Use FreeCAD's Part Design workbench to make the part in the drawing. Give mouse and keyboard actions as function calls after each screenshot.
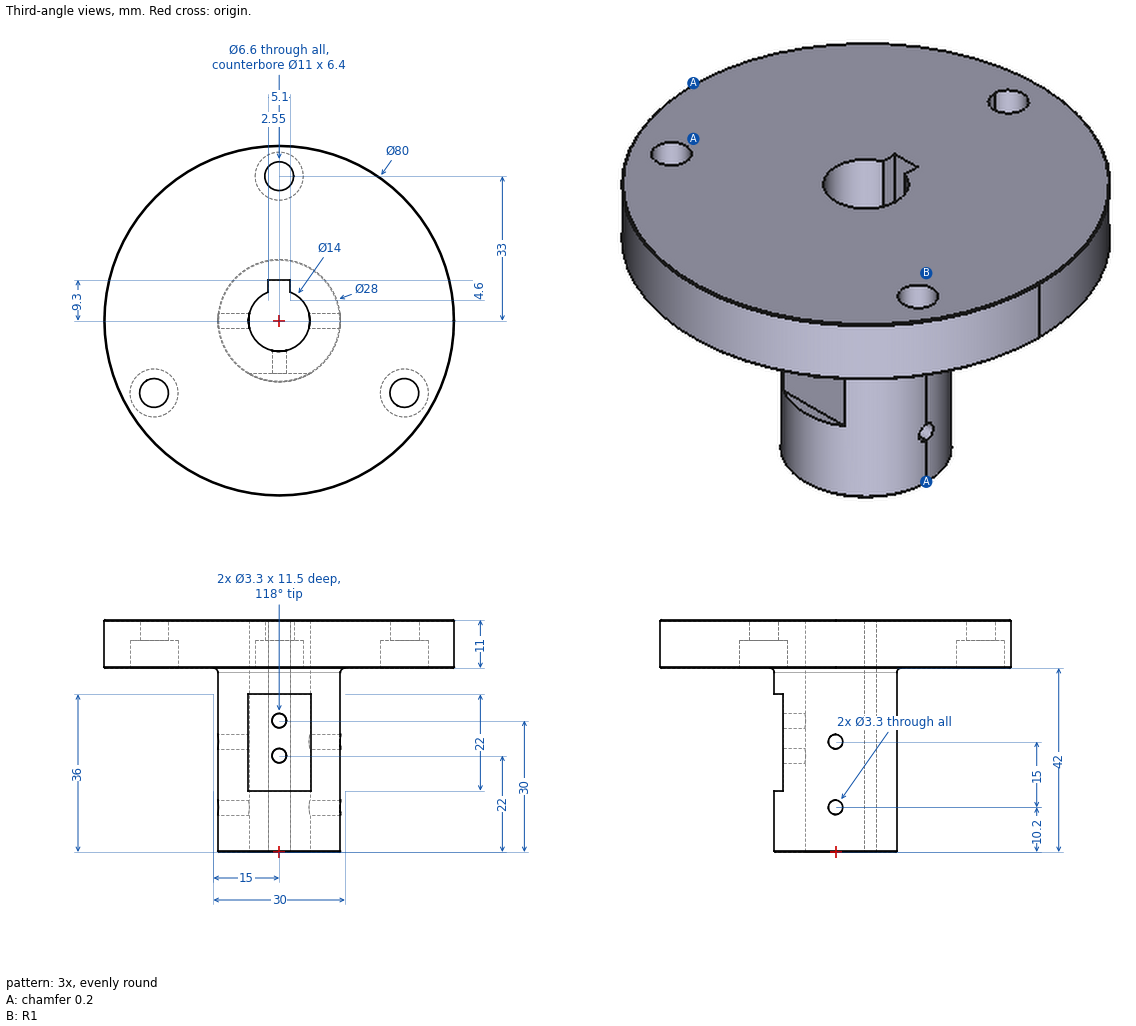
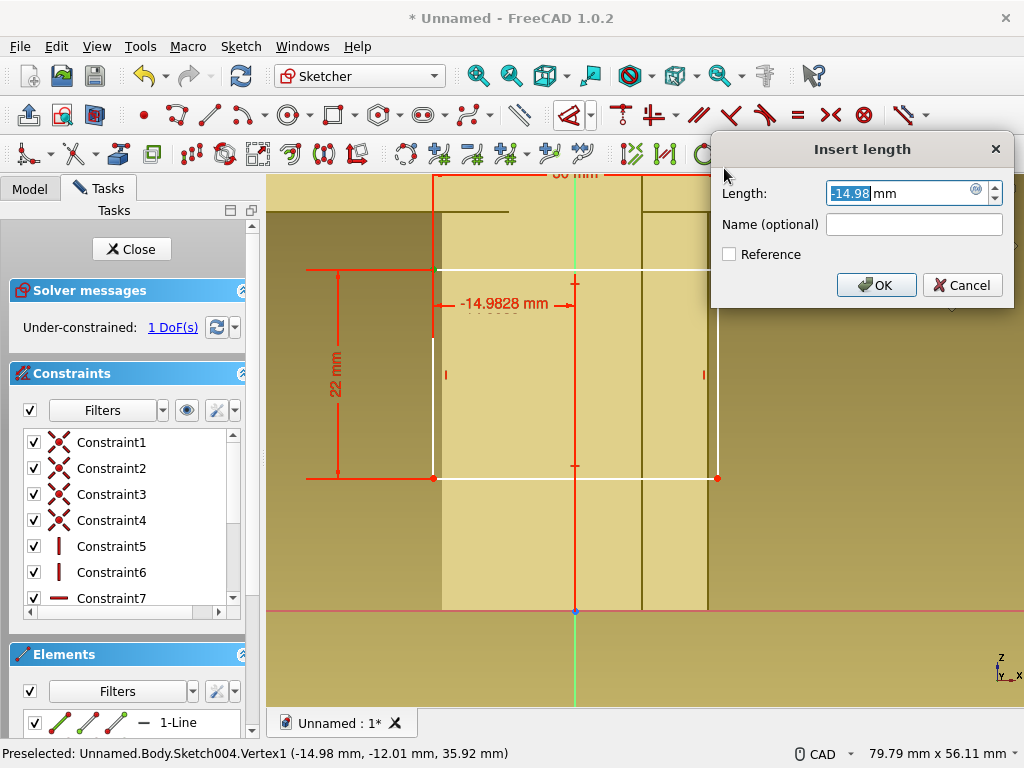
text(-15)
key(Return)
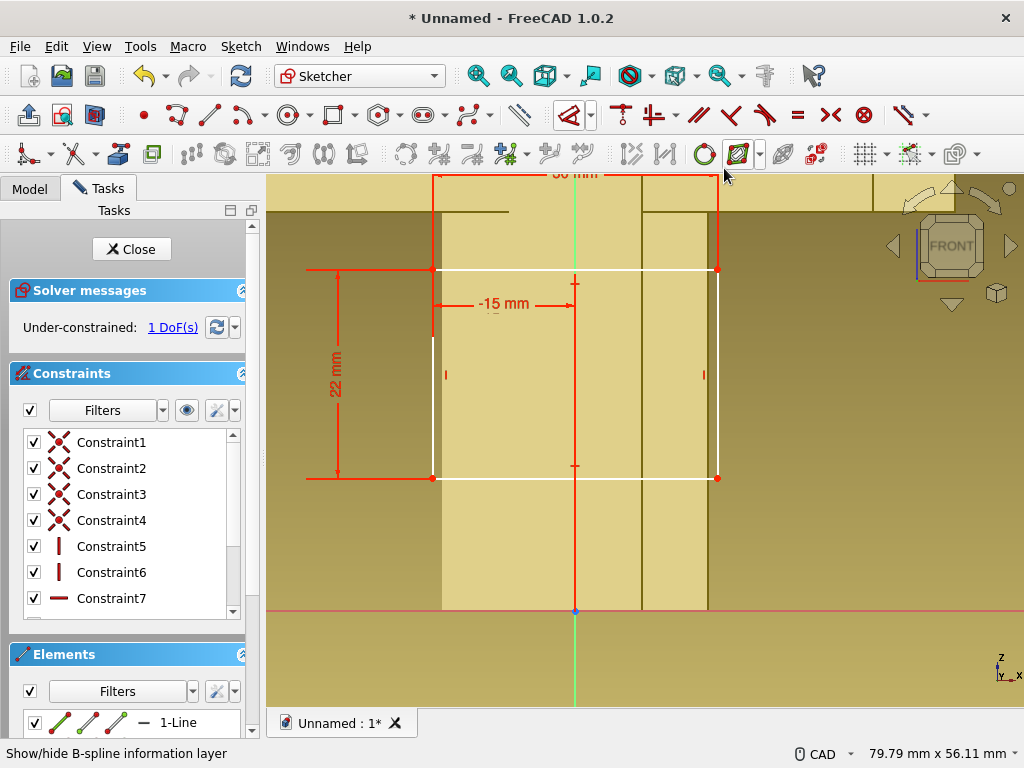
click(433, 270)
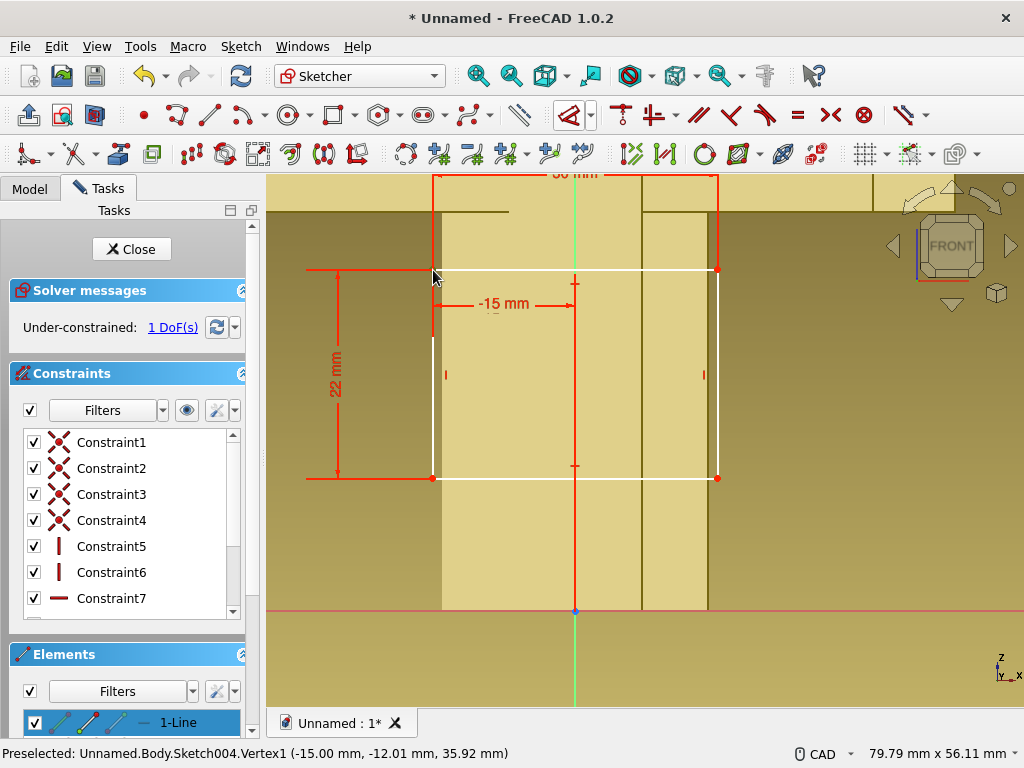
key(i)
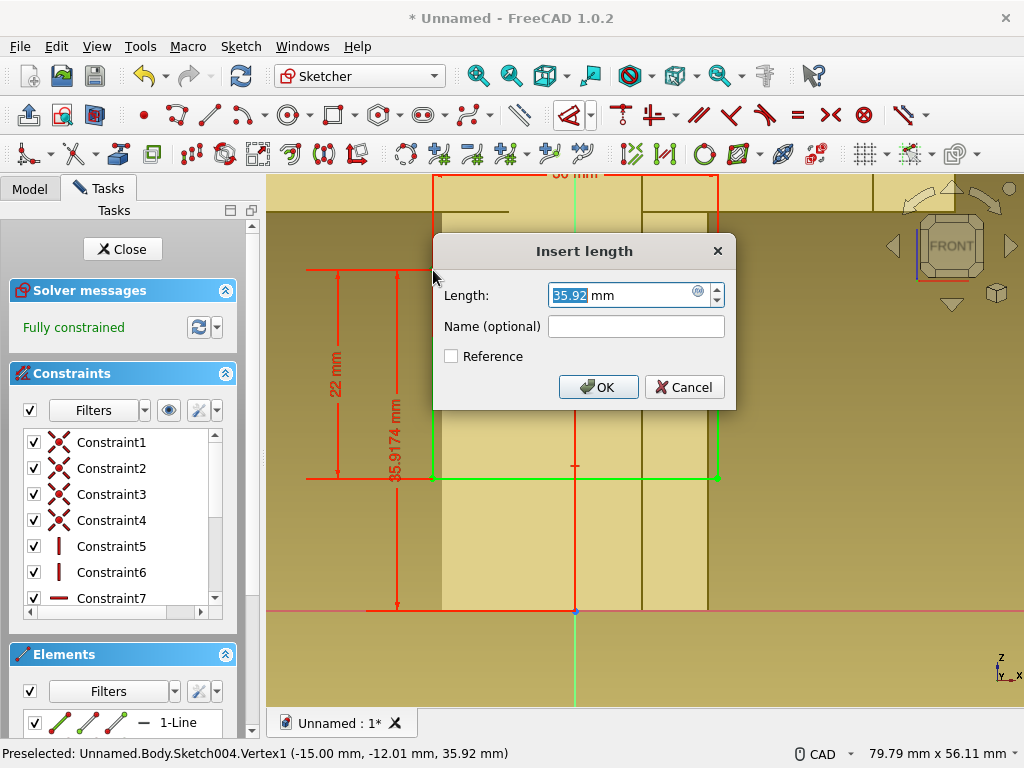
text(36)
key(Return)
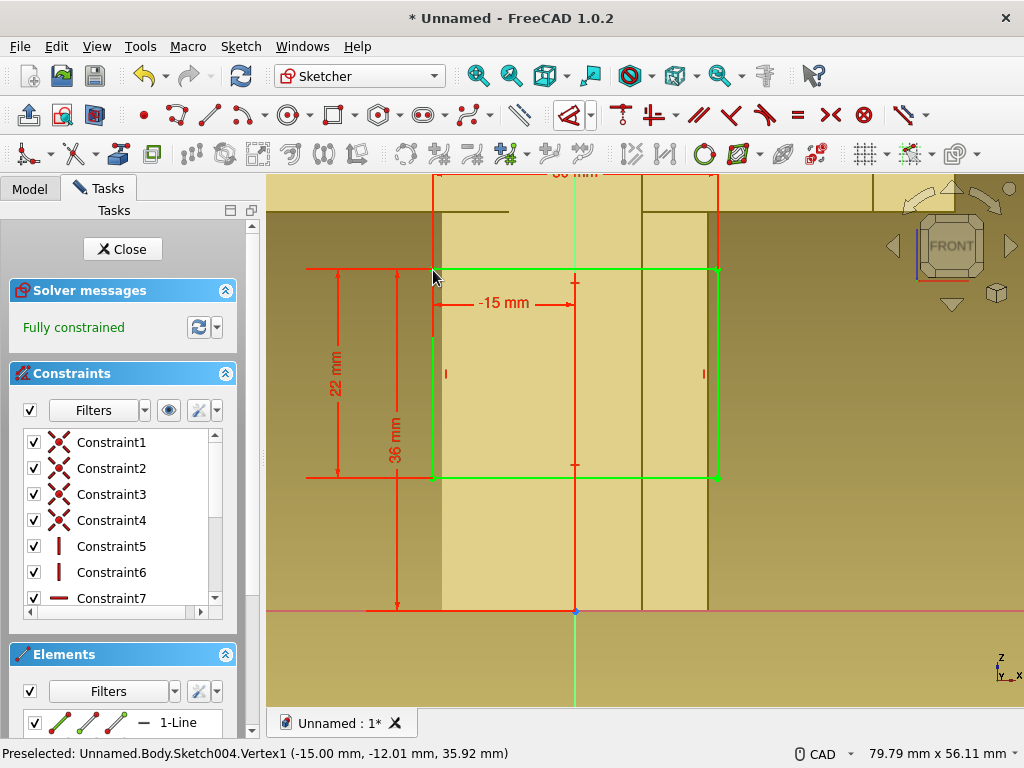
click(123, 249)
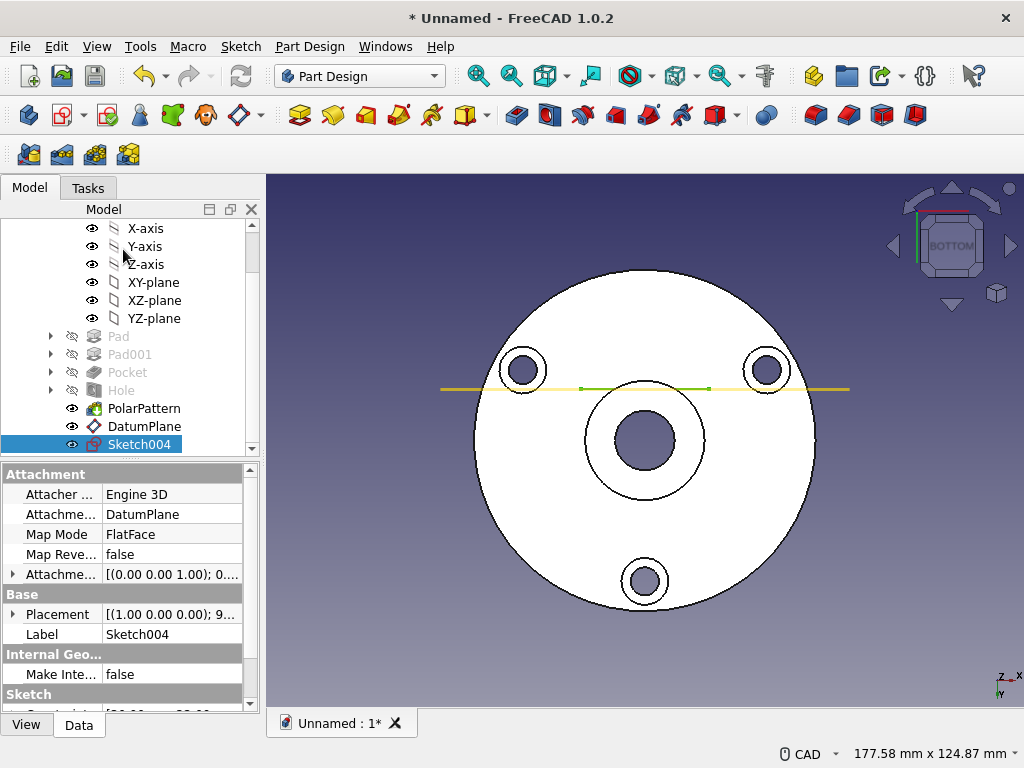
click(517, 116)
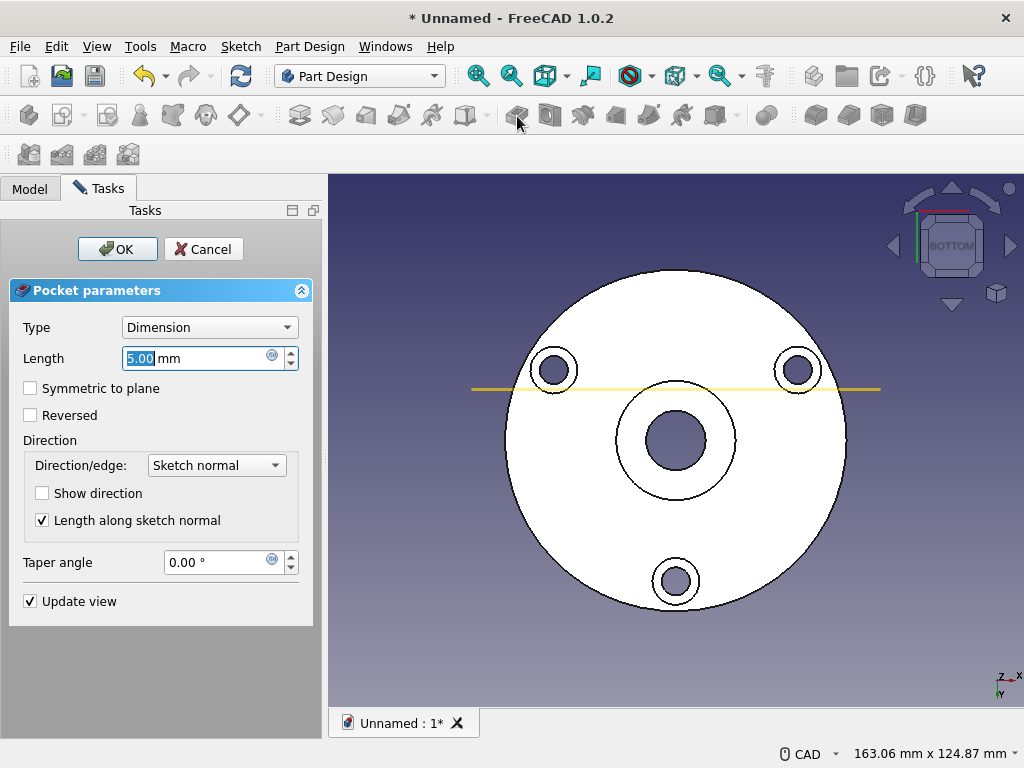
click(210, 328)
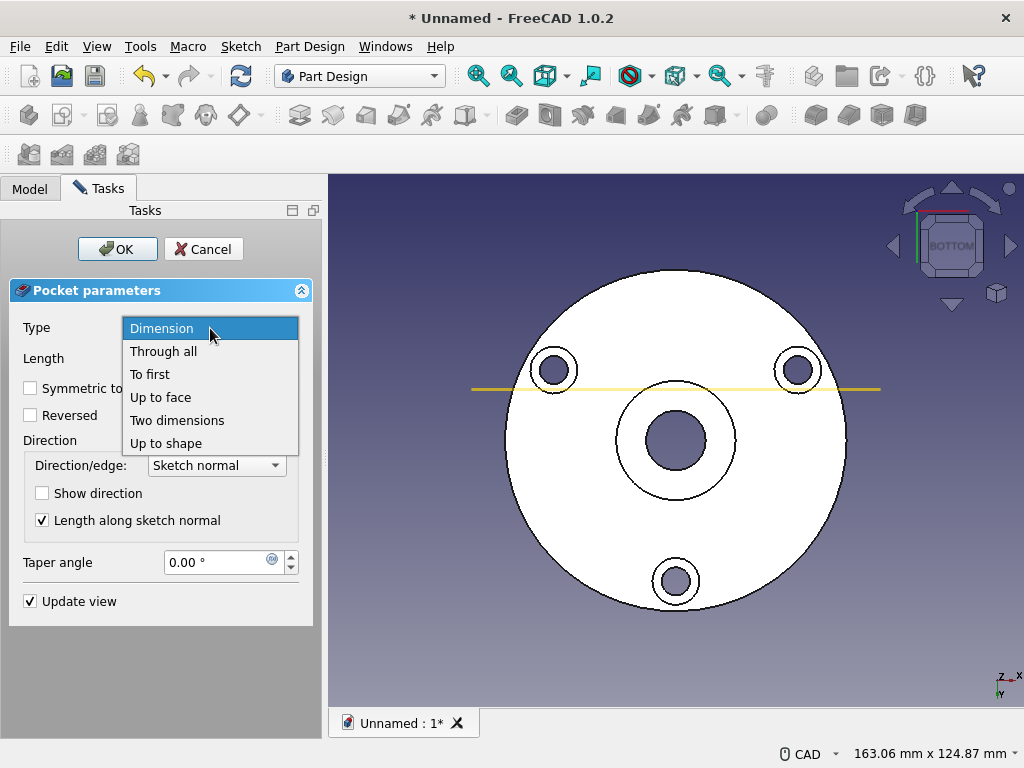
click(208, 352)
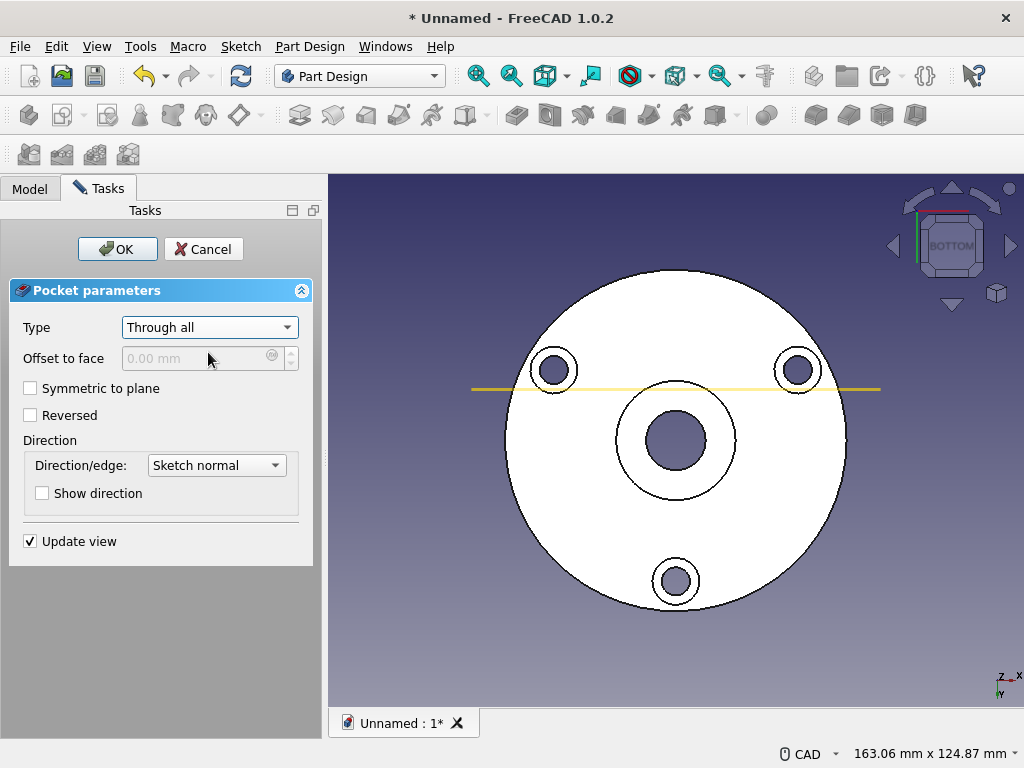
click(31, 415)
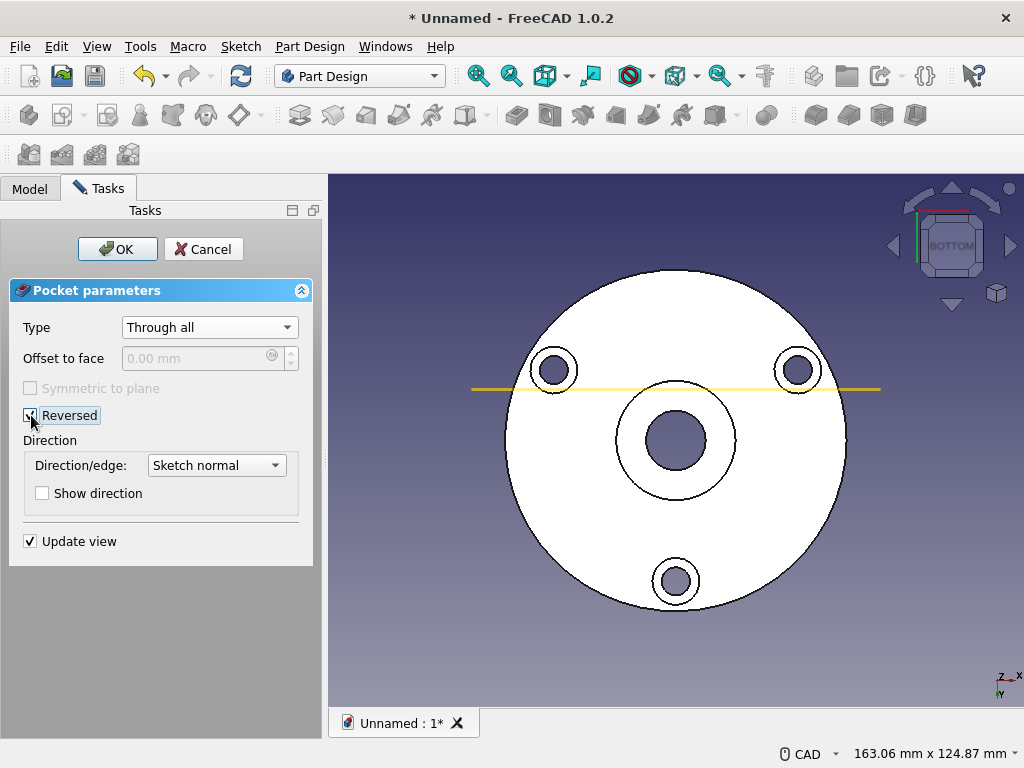
click(118, 249)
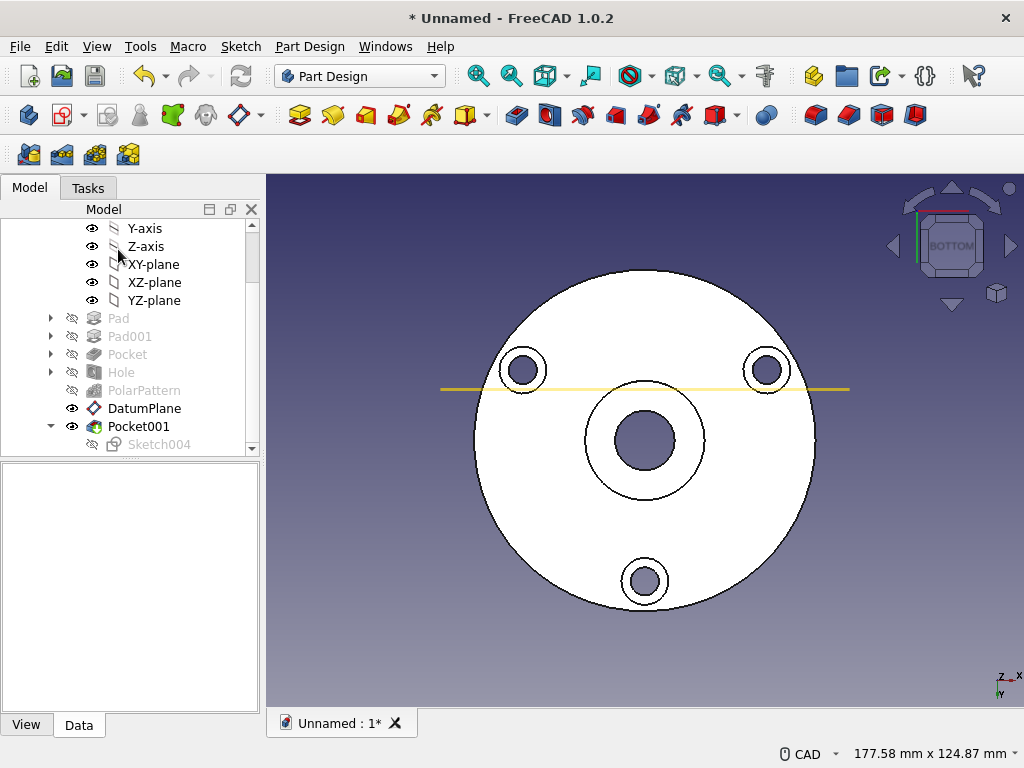
click(117, 408)
key(space)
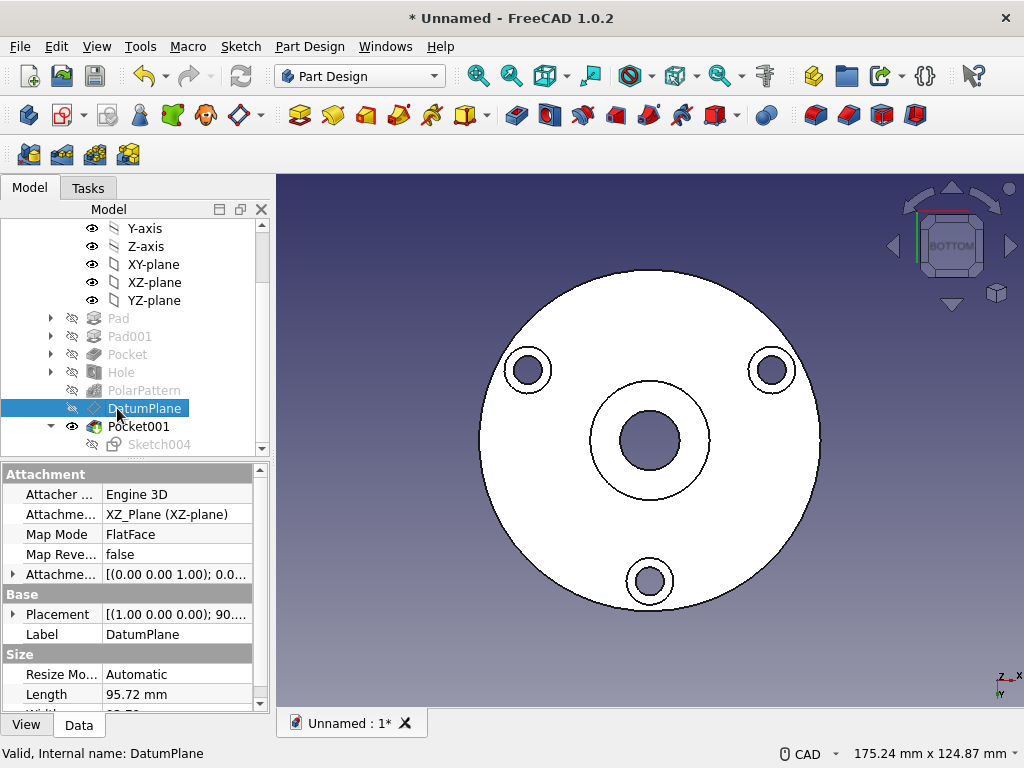
key(0)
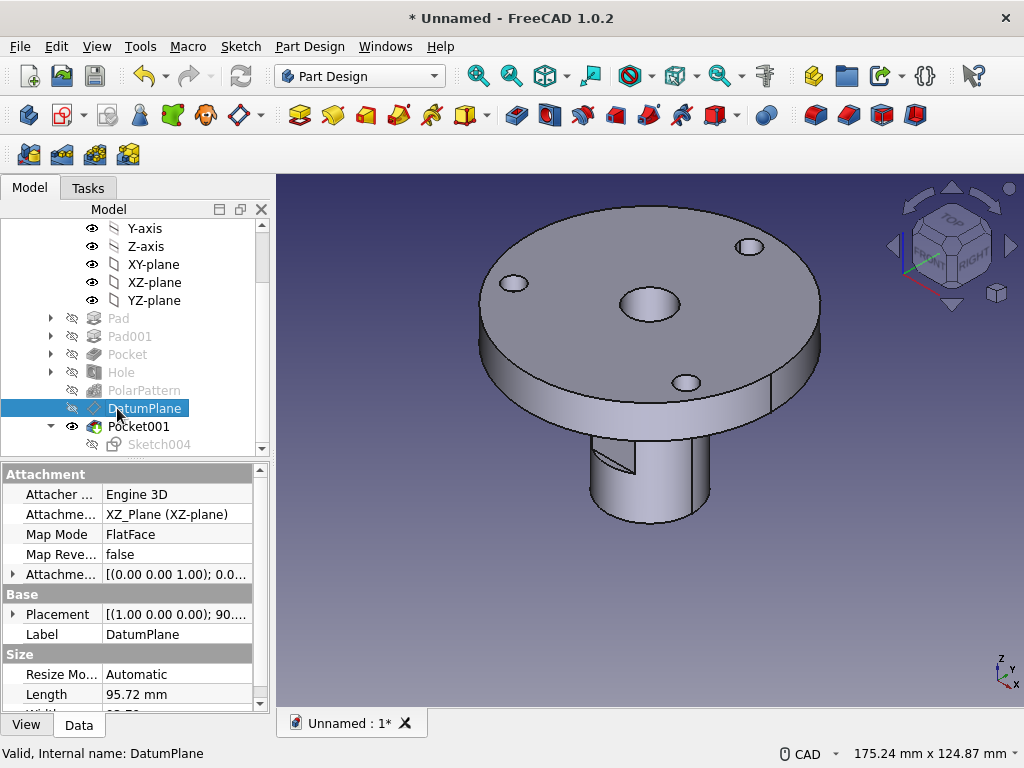
key(v)
key(f)